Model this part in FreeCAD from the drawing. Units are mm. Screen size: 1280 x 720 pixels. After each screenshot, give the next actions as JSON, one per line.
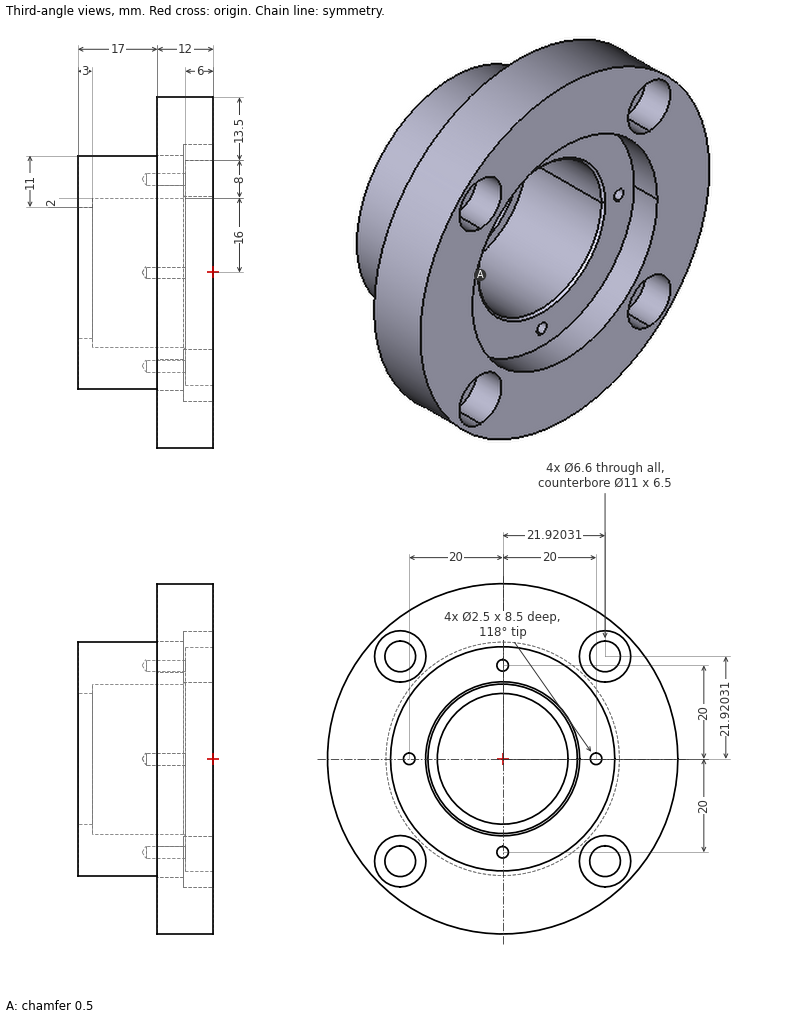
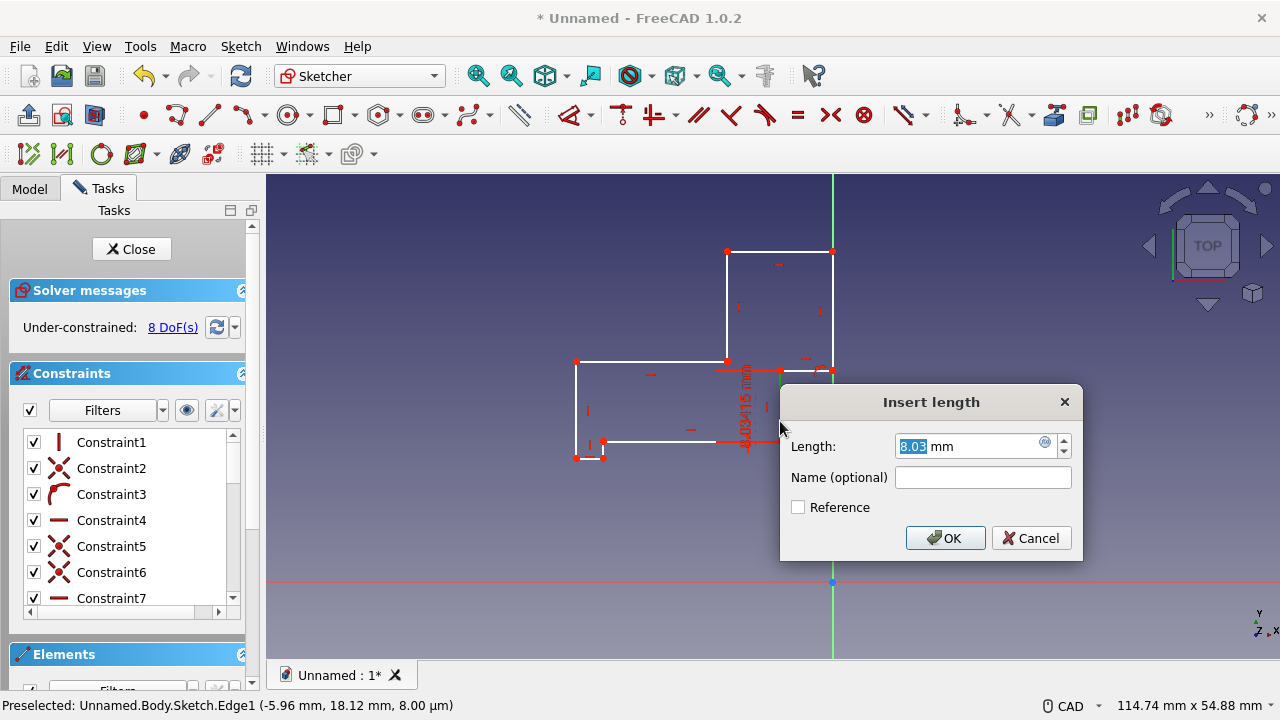
{"action": "type", "text": "8"}
{"action": "key", "text": "Return"}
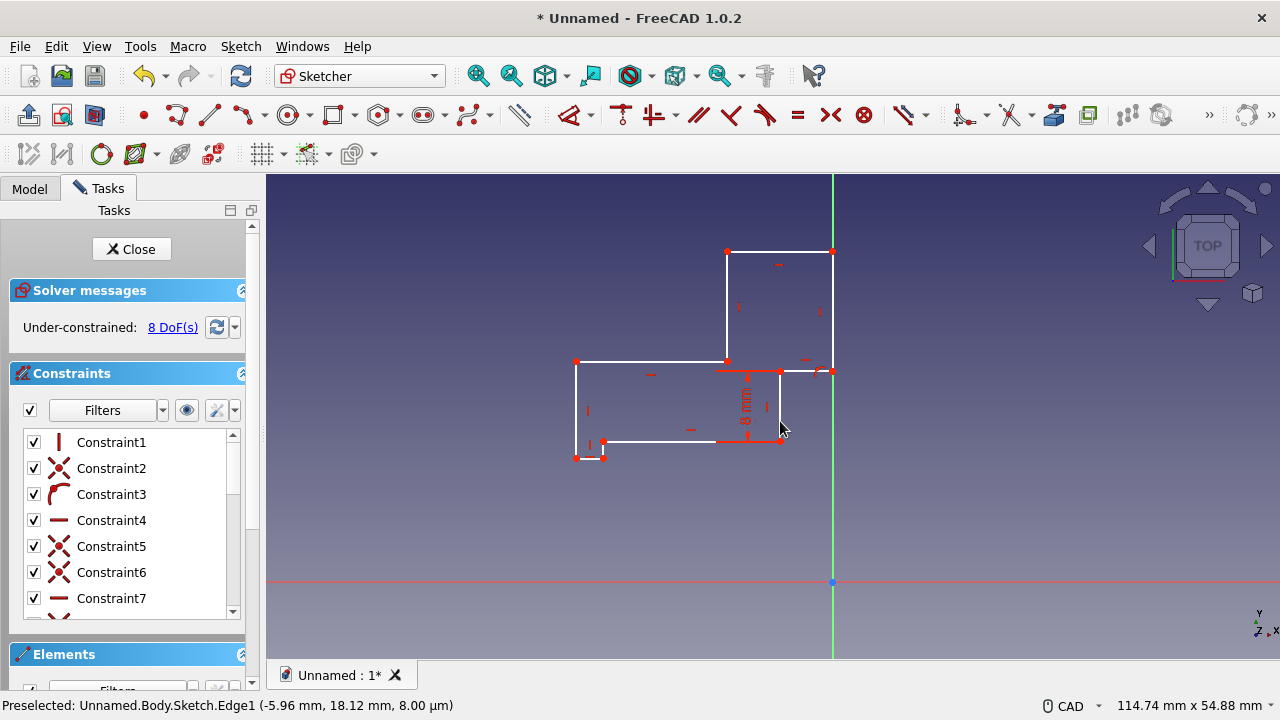
{"action": "left_click", "coordinate": [796, 371]}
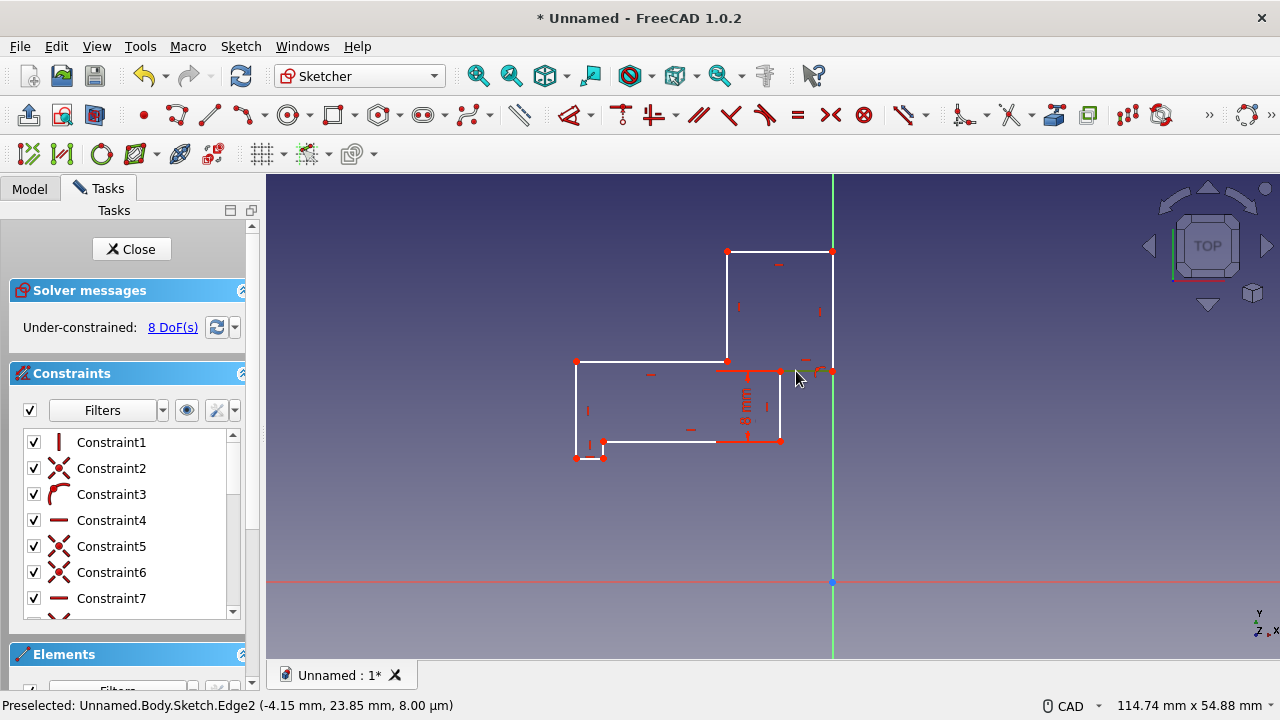
{"action": "key", "text": "l"}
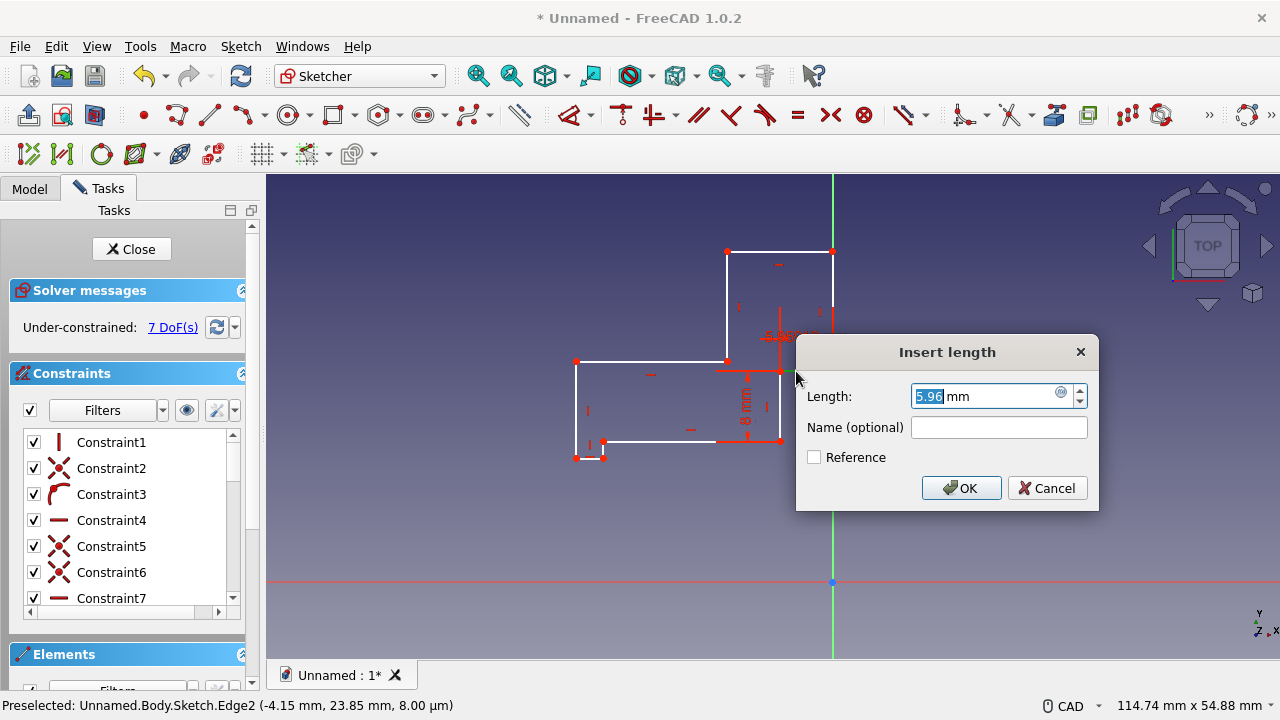
{"action": "type", "text": "6"}
{"action": "key", "text": "Return"}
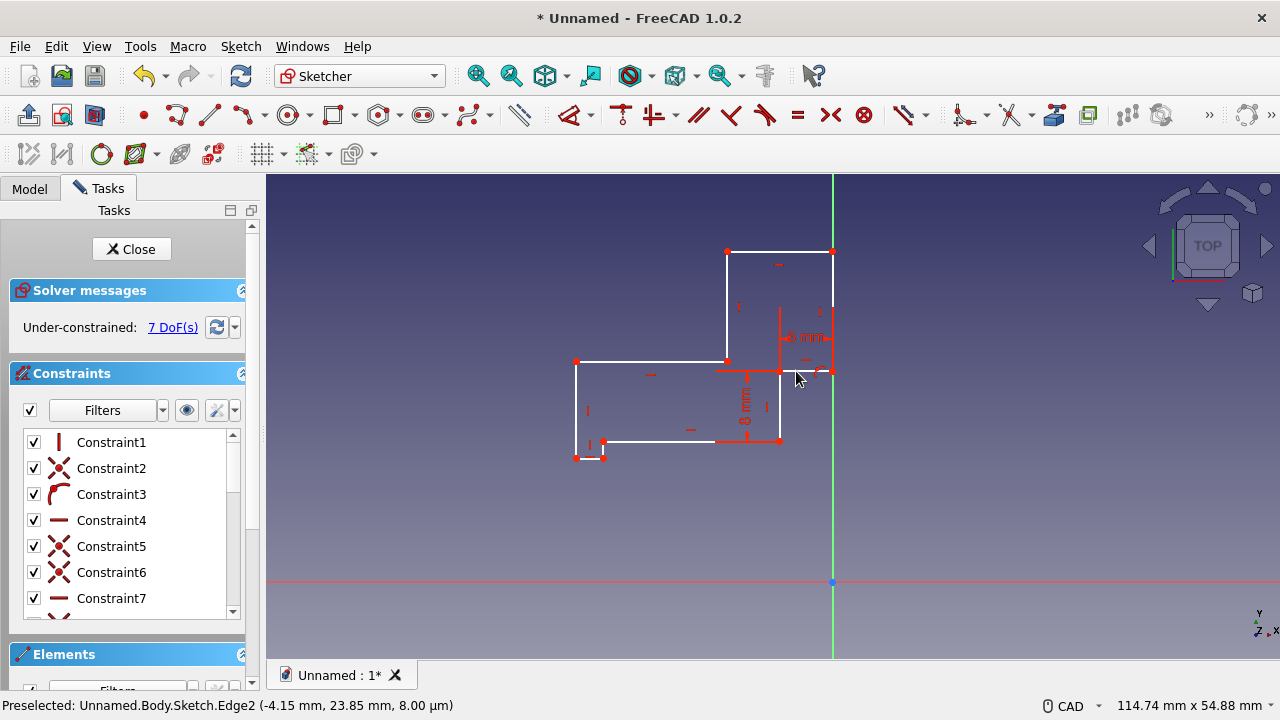
{"action": "scroll", "coordinate": [587, 459], "scroll_direction": "up", "scroll_amount": 3}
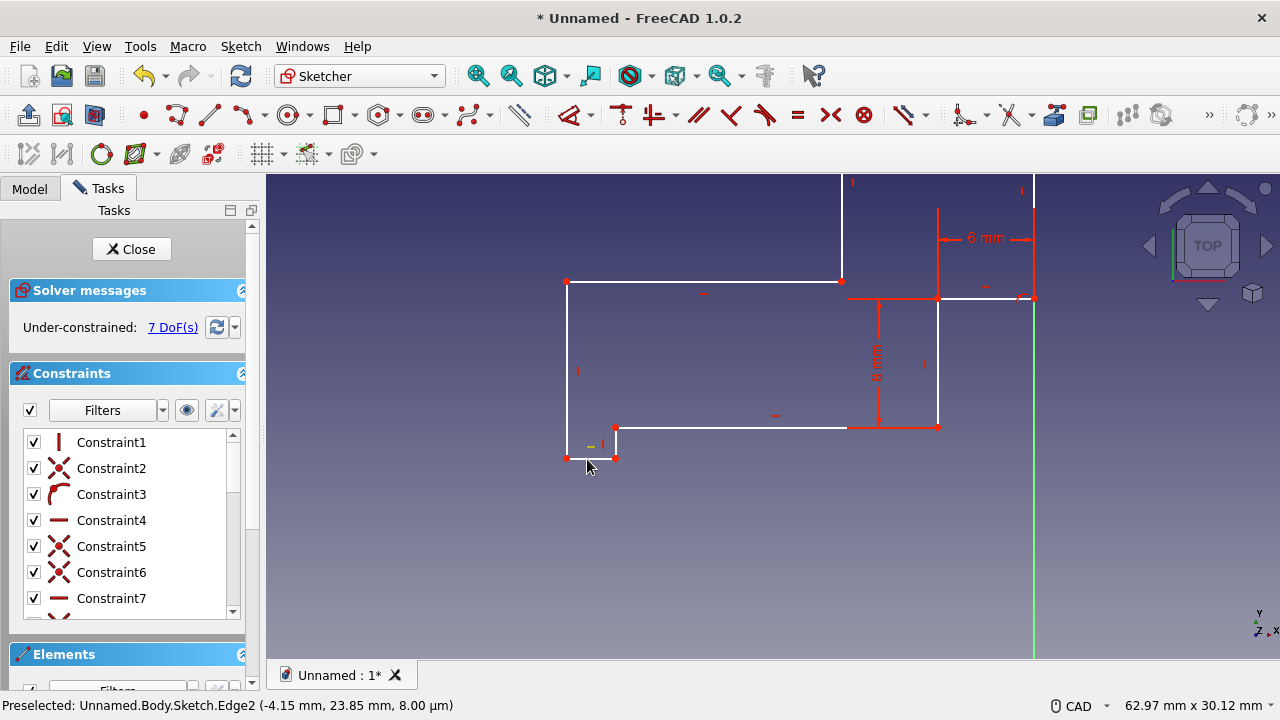
{"action": "left_click", "coordinate": [586, 459]}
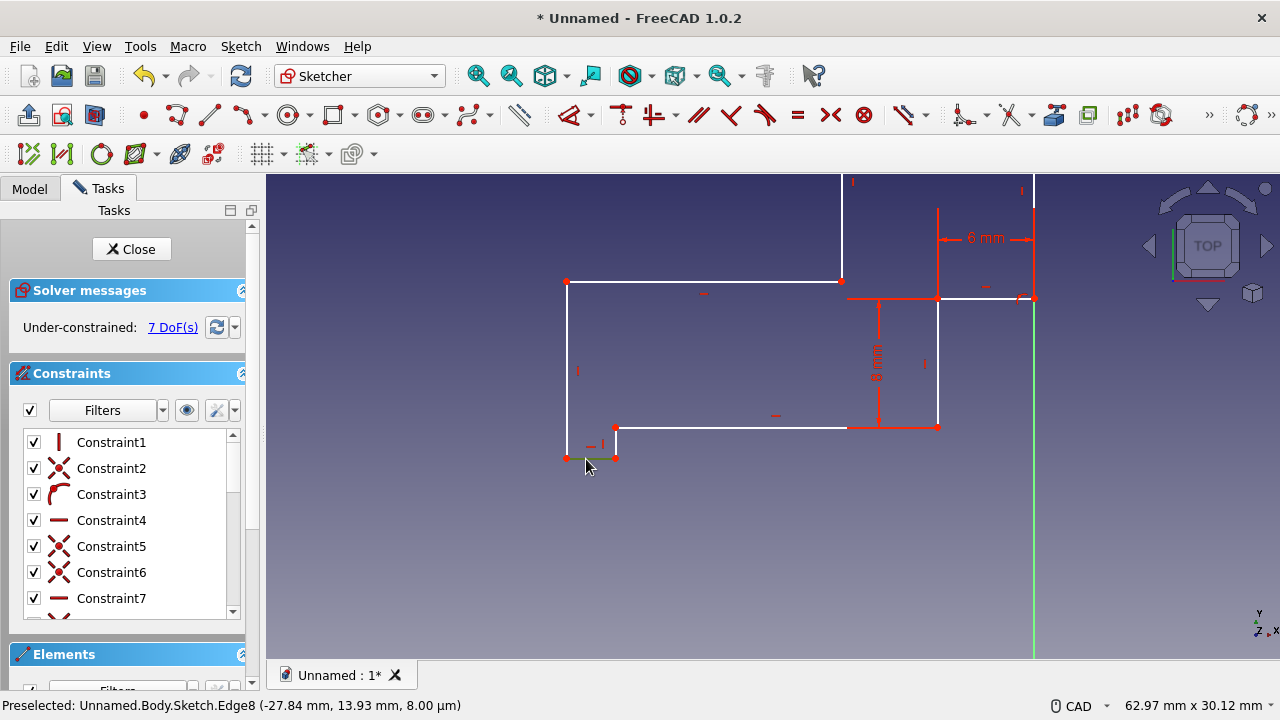
{"action": "left_click", "coordinate": [590, 116]}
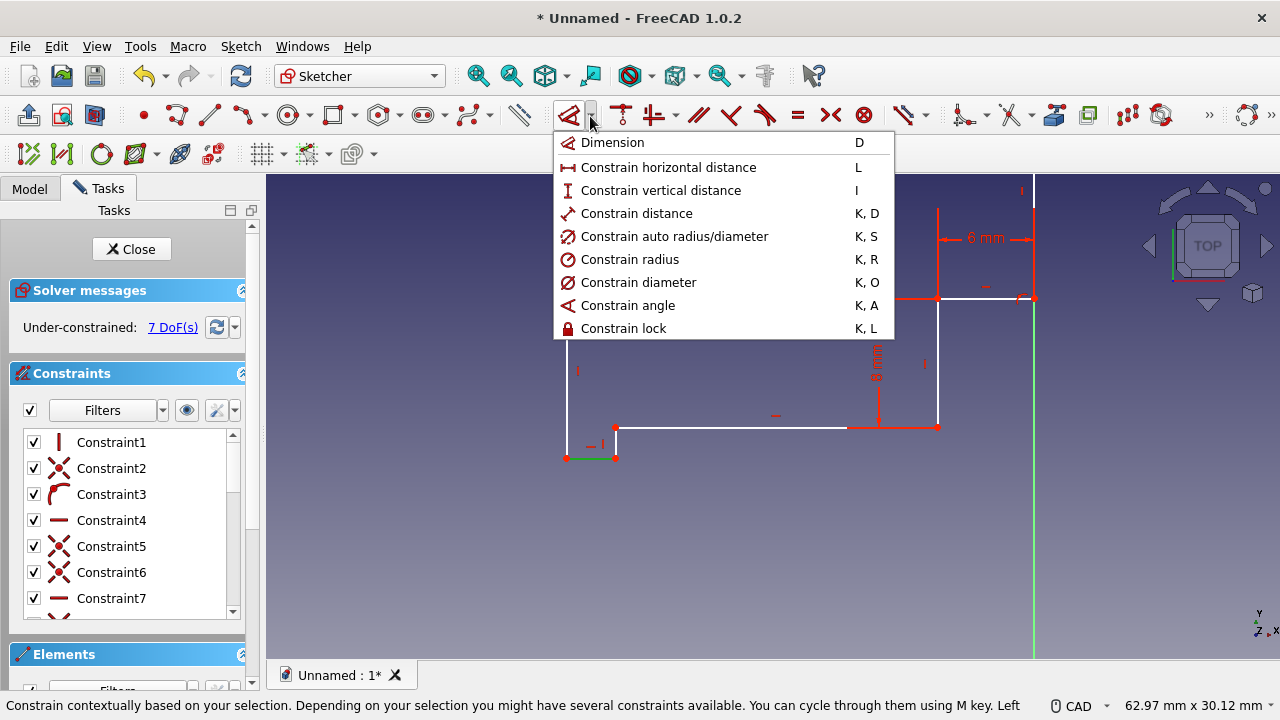
{"action": "left_click", "coordinate": [724, 168]}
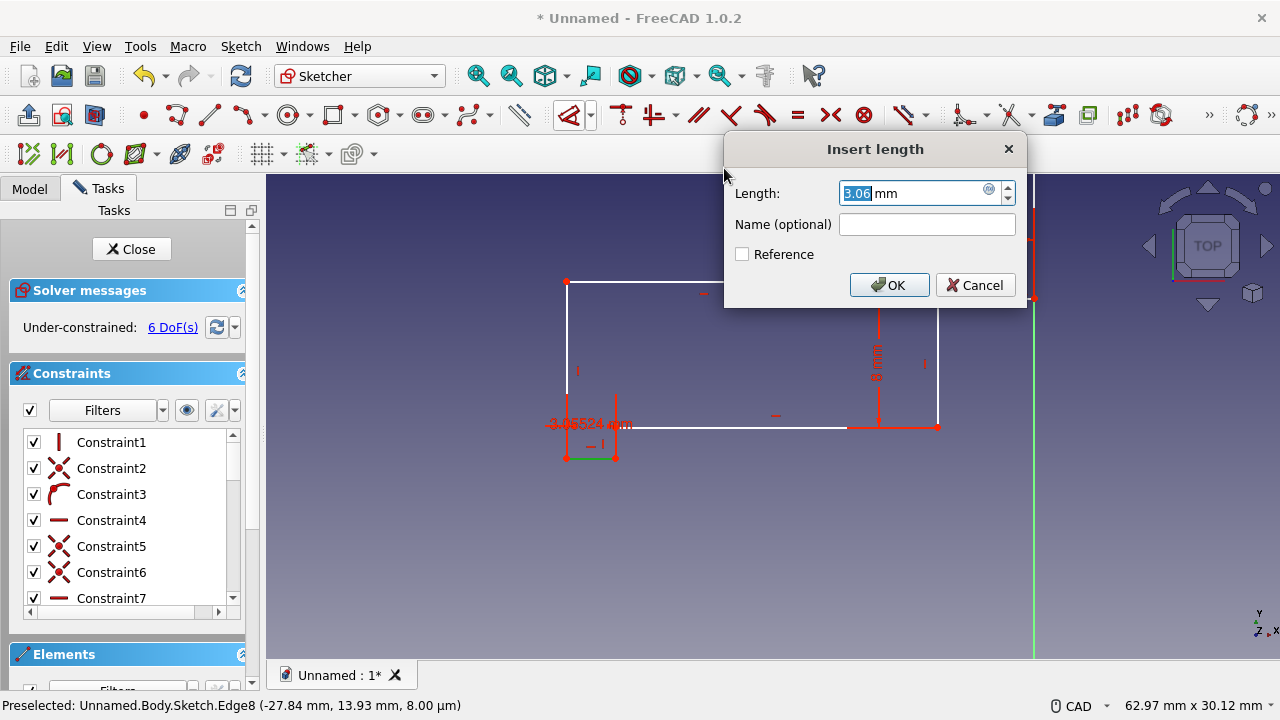
{"action": "type", "text": "3"}
{"action": "key", "text": "Return"}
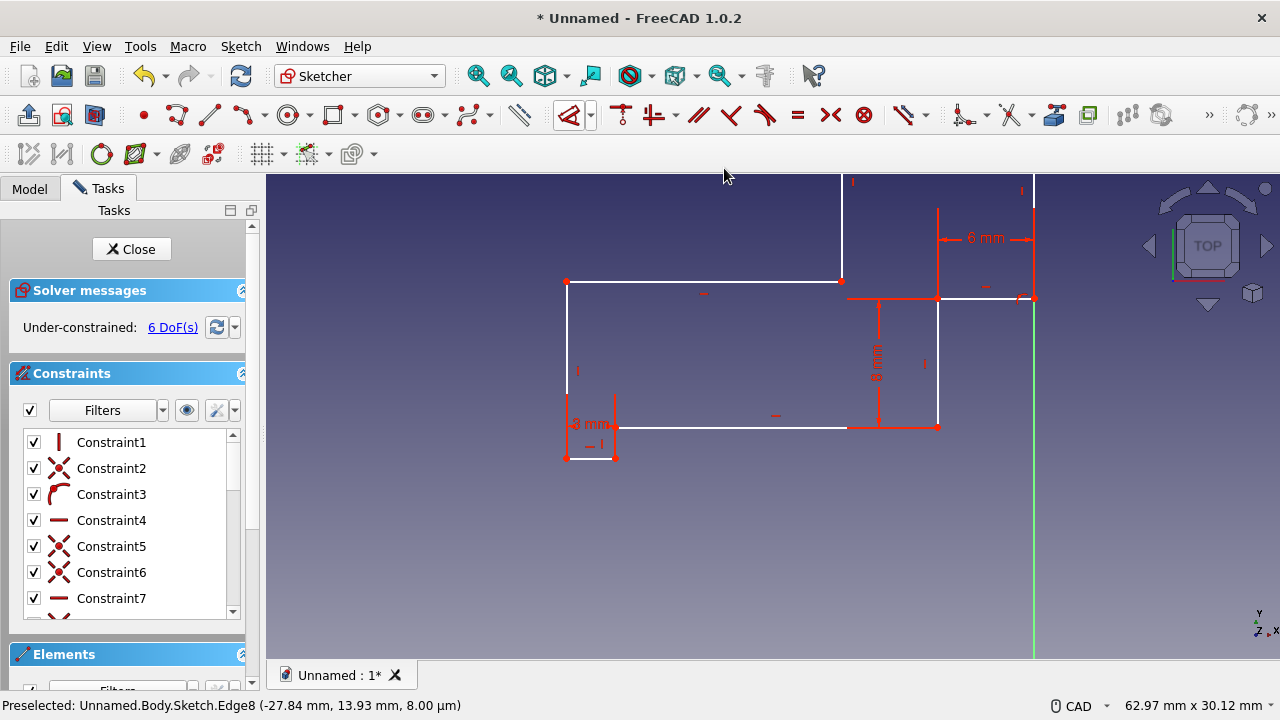
{"action": "scroll", "coordinate": [615, 449], "scroll_direction": "up", "scroll_amount": 2}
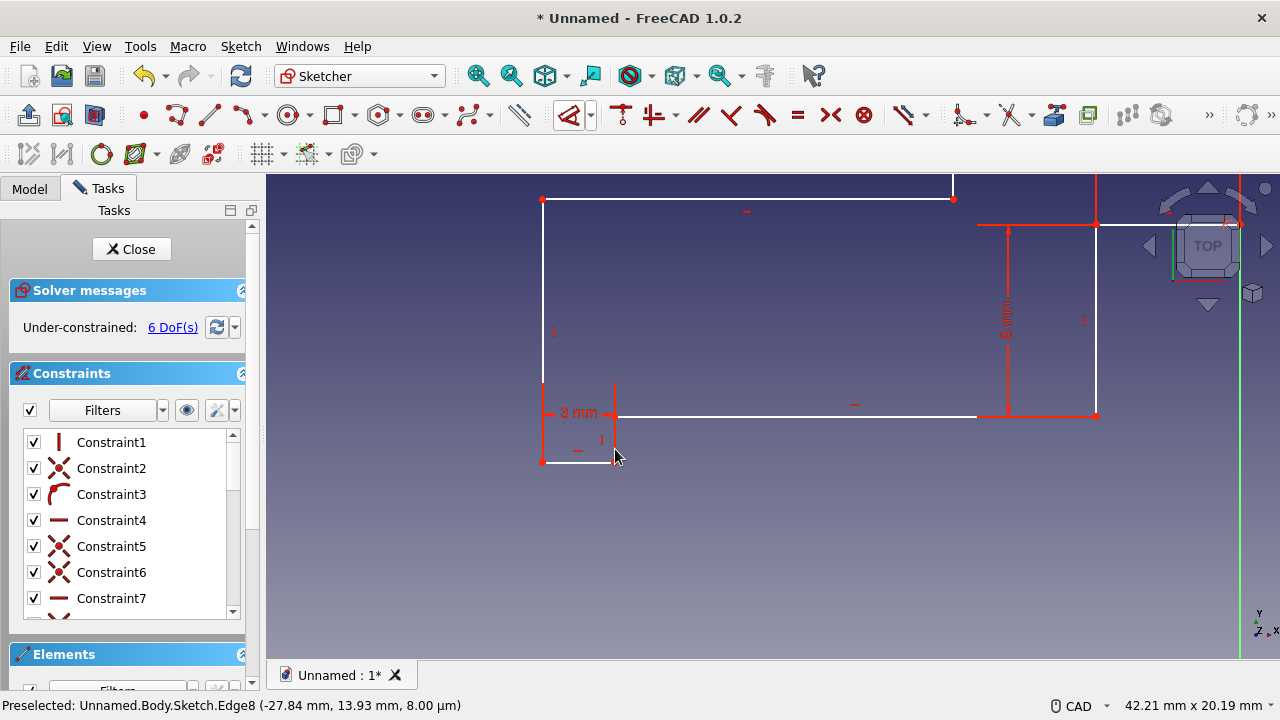
{"action": "left_click", "coordinate": [615, 449]}